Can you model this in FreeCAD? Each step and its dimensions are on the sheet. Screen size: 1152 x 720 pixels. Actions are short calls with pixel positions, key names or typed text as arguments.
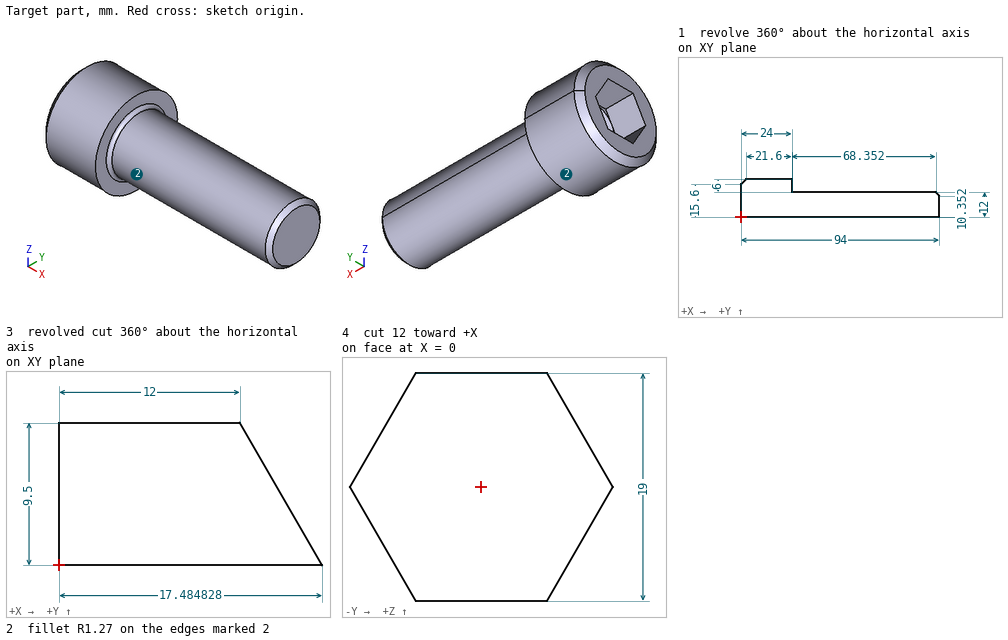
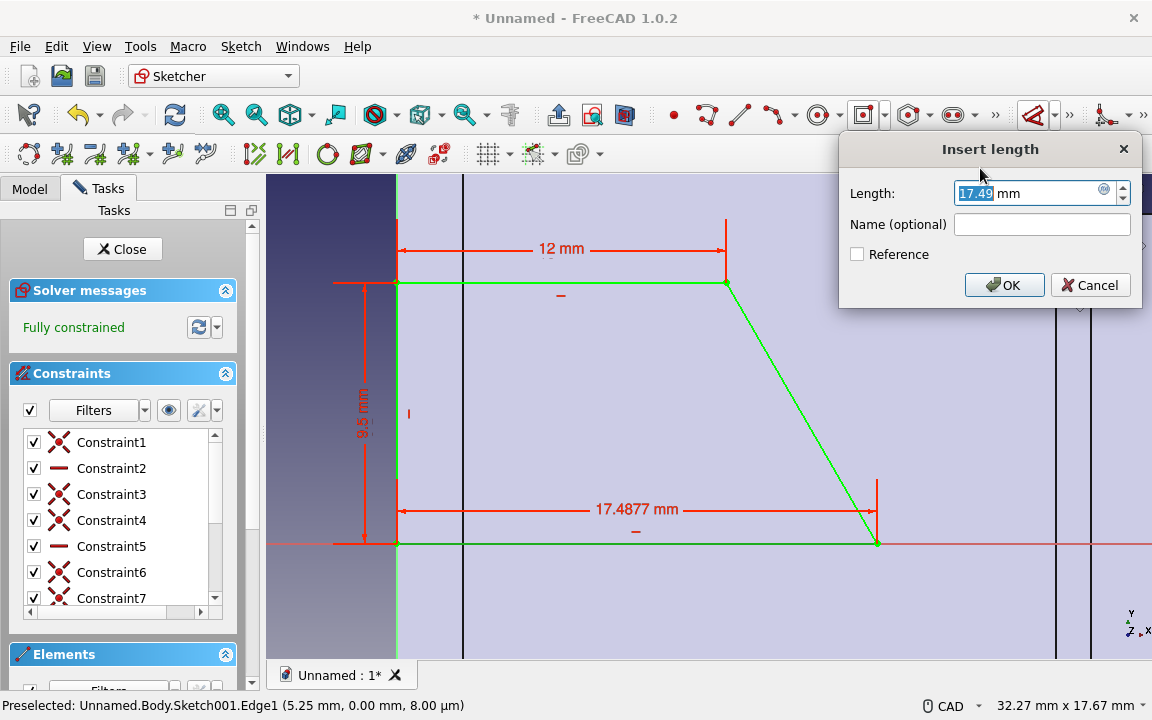
text(17.484828)
key(Return)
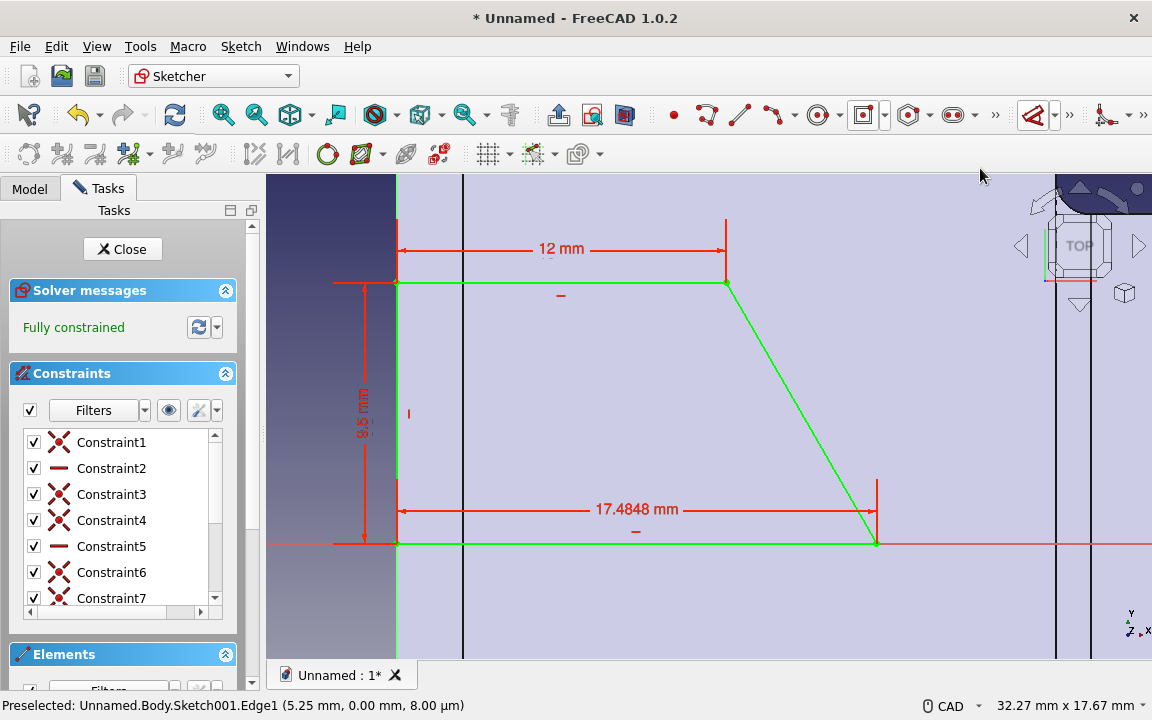
click(123, 249)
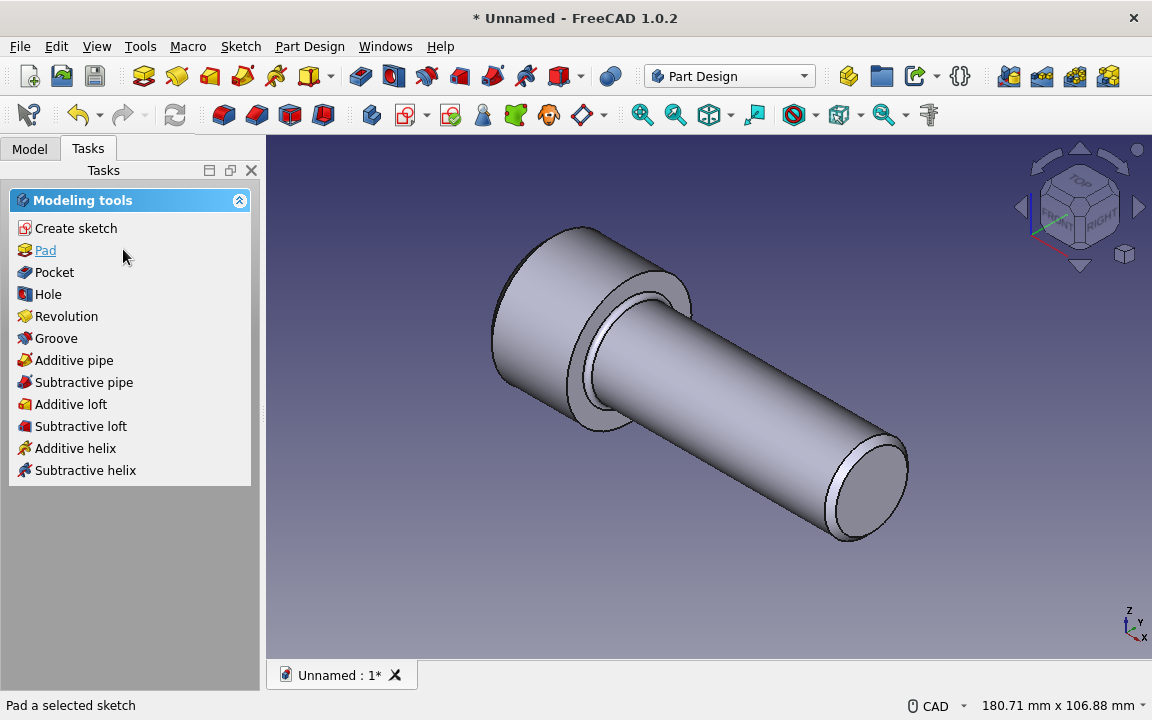
click(427, 76)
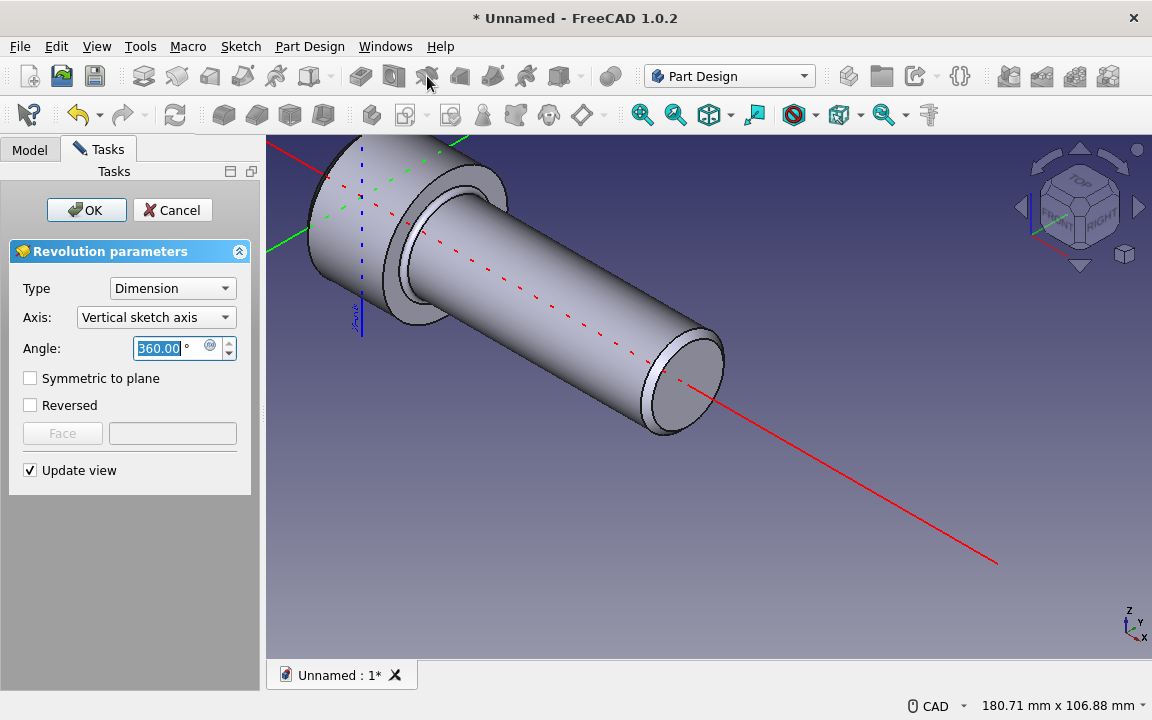
click(157, 318)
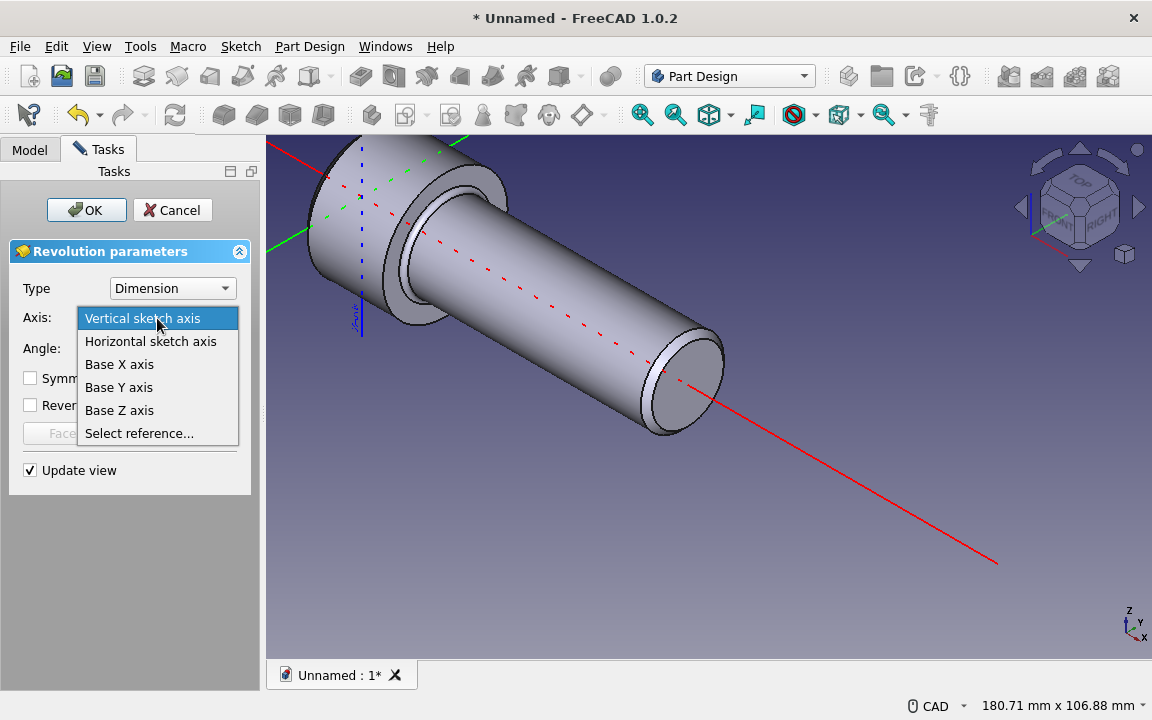
click(156, 342)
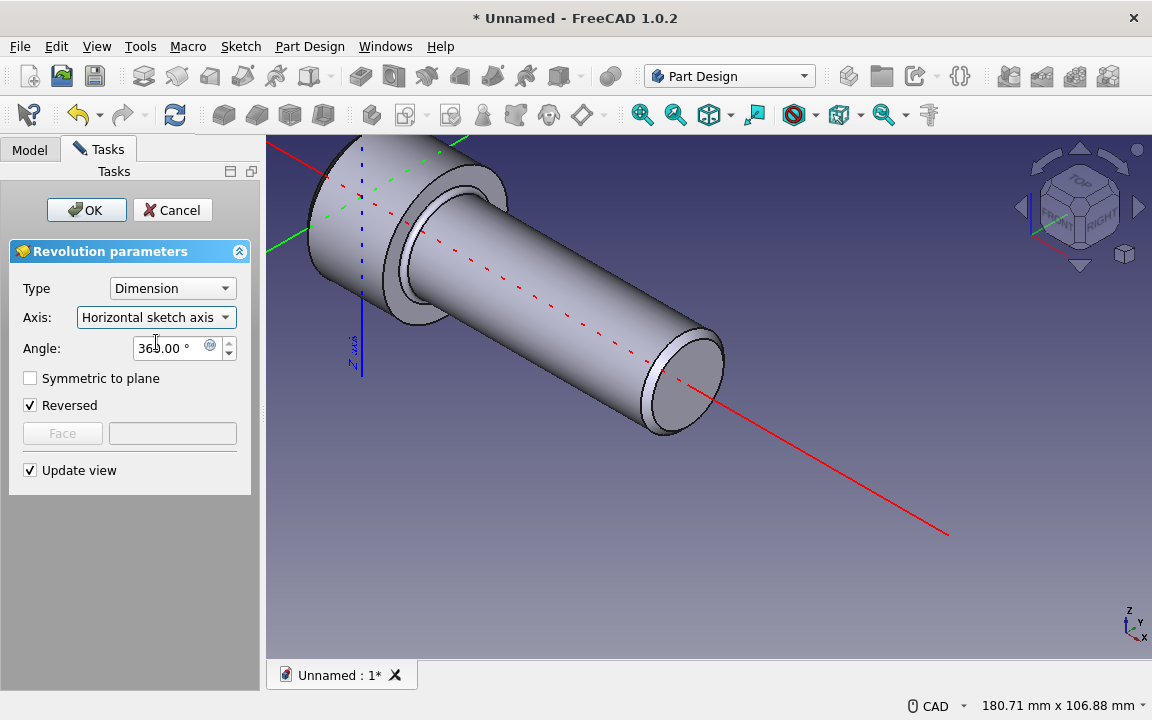
click(87, 210)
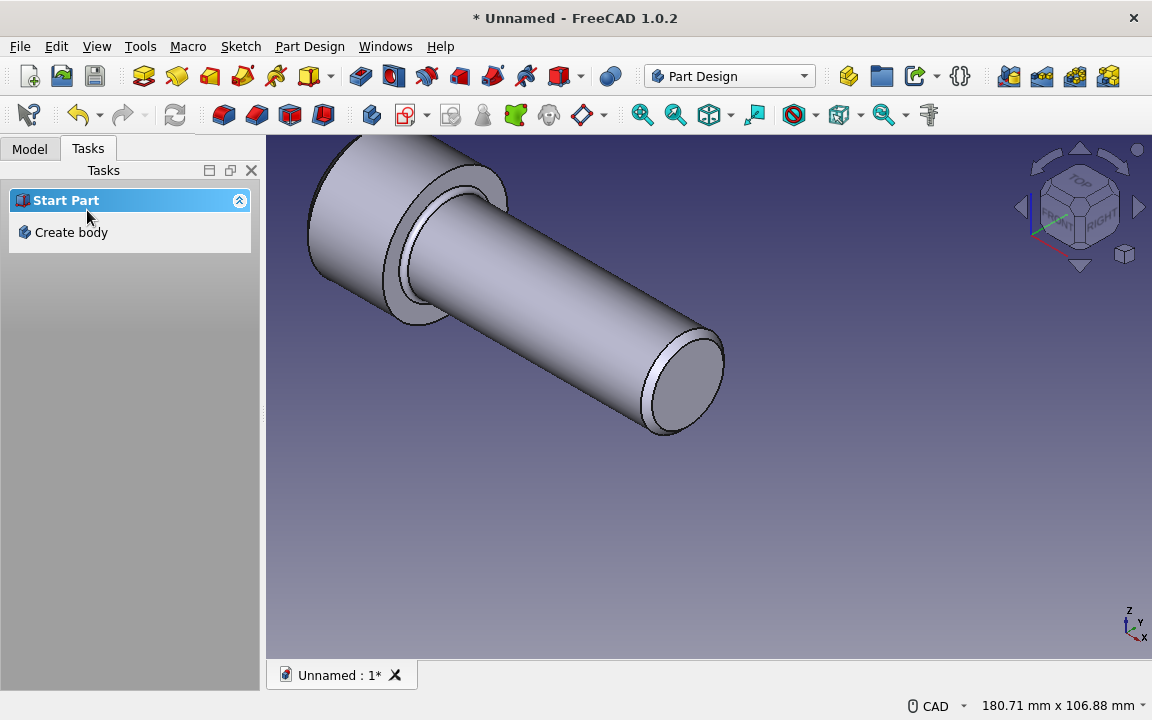
click(643, 116)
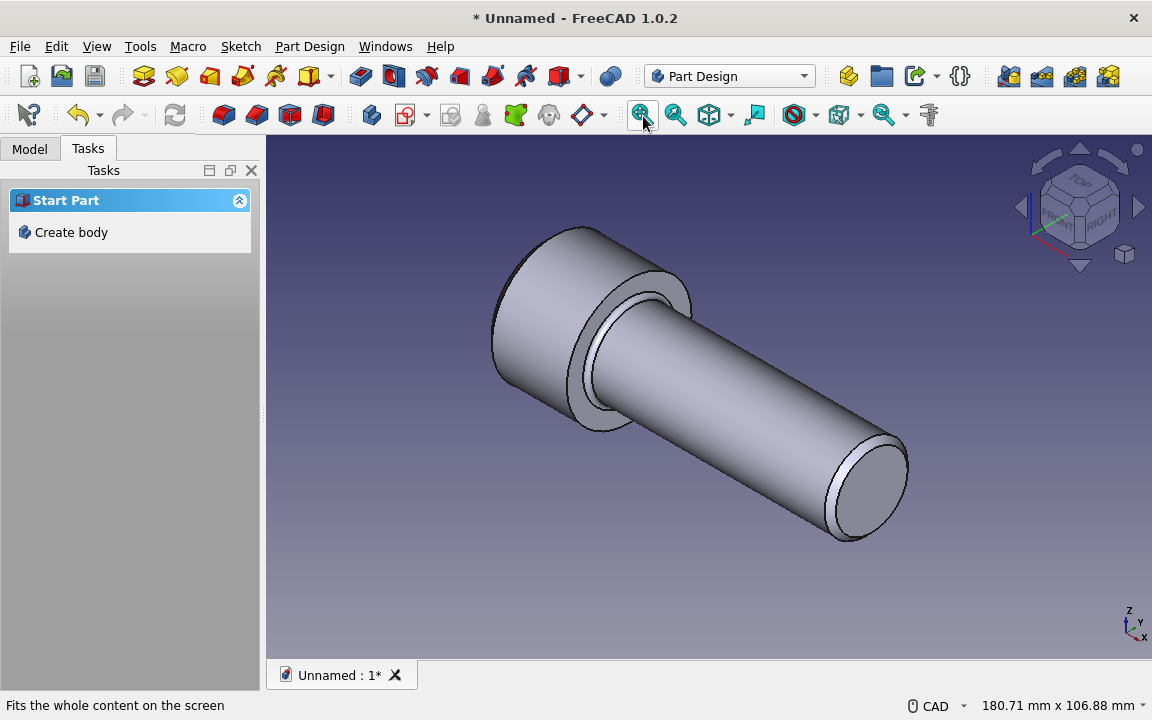
key(6)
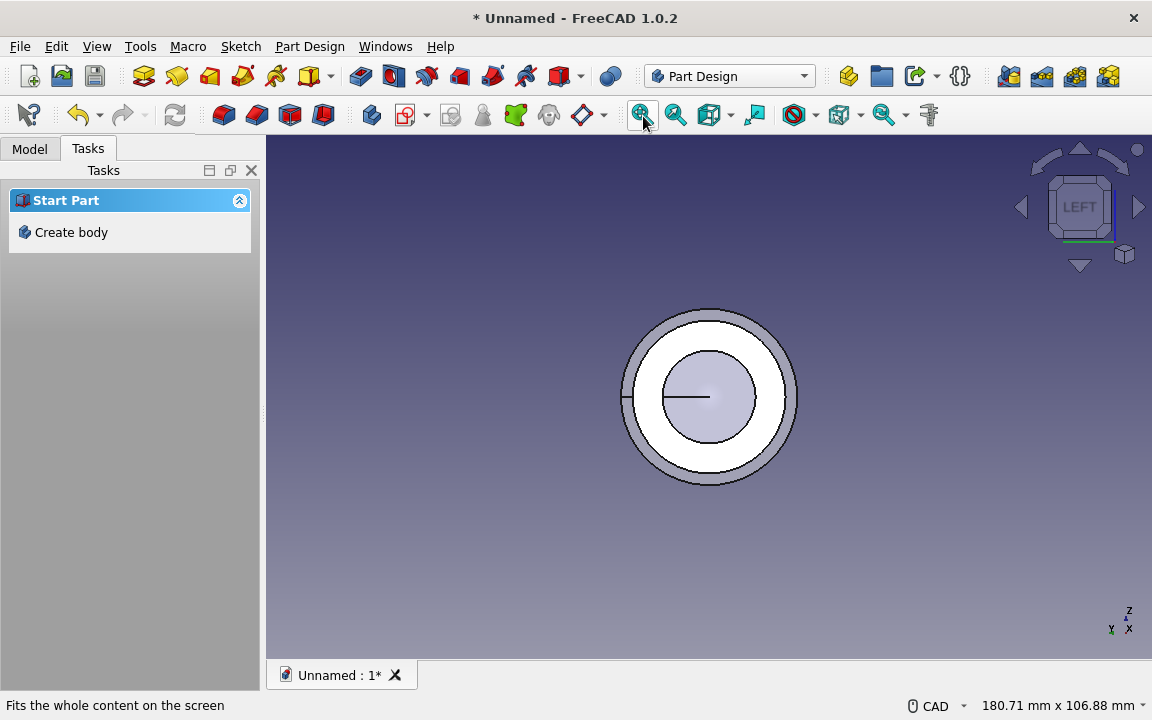
click(643, 116)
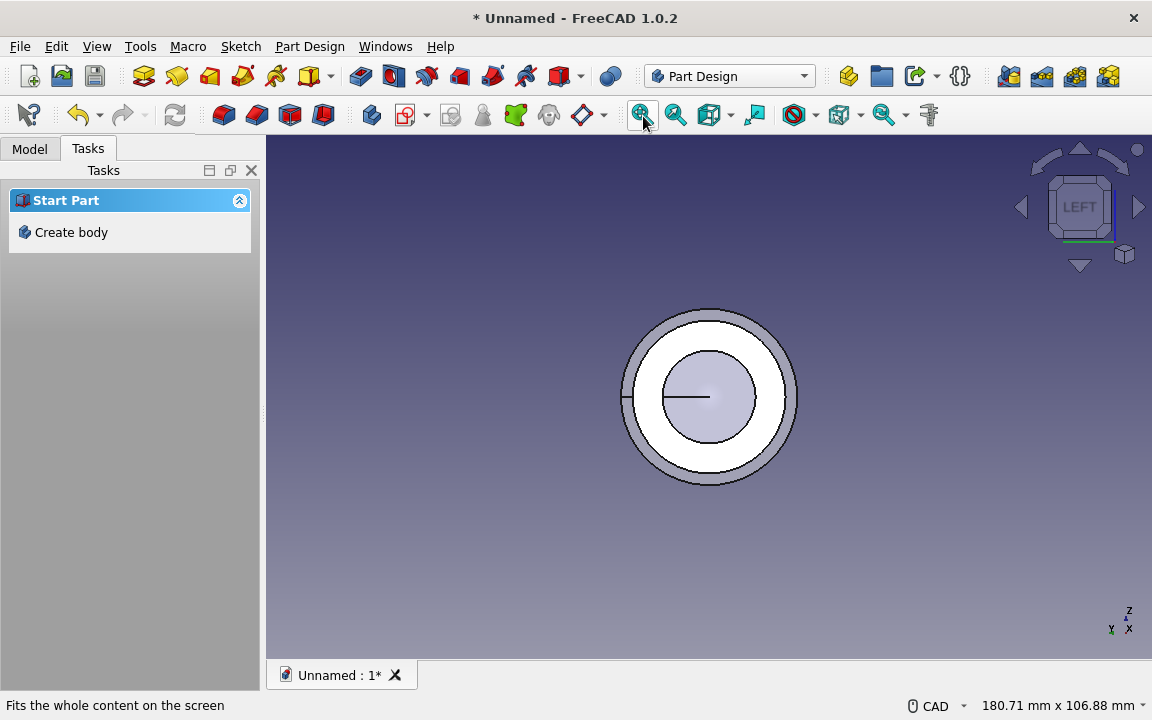
click(665, 352)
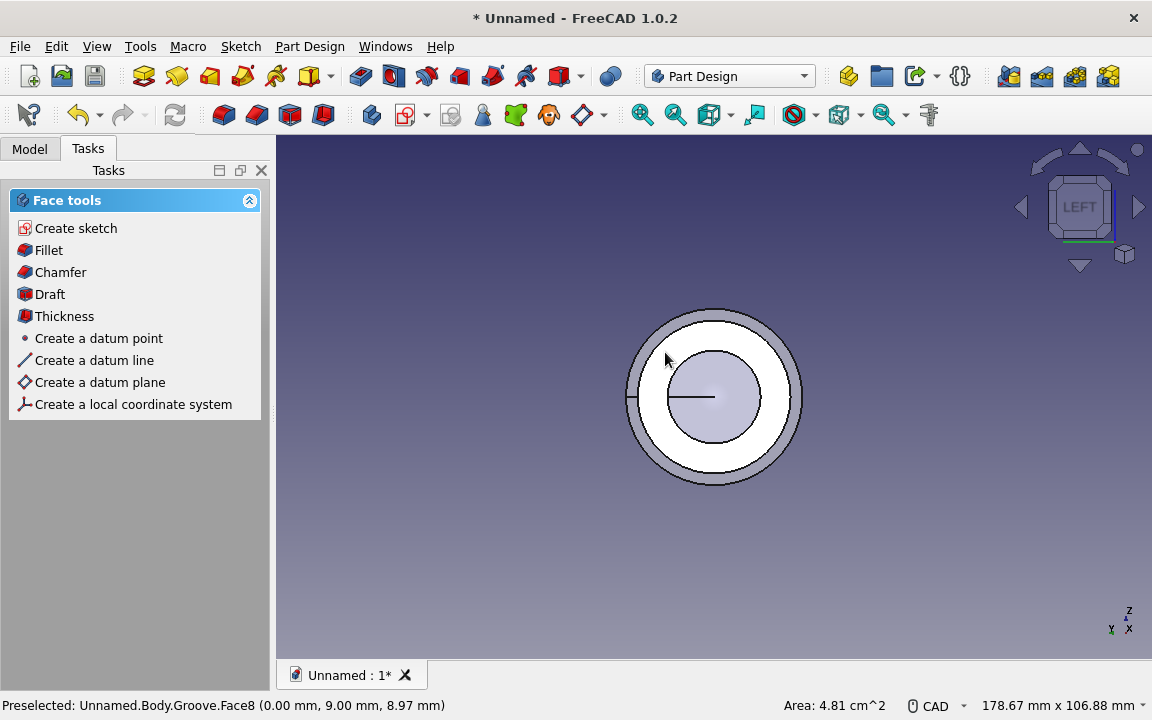
click(404, 116)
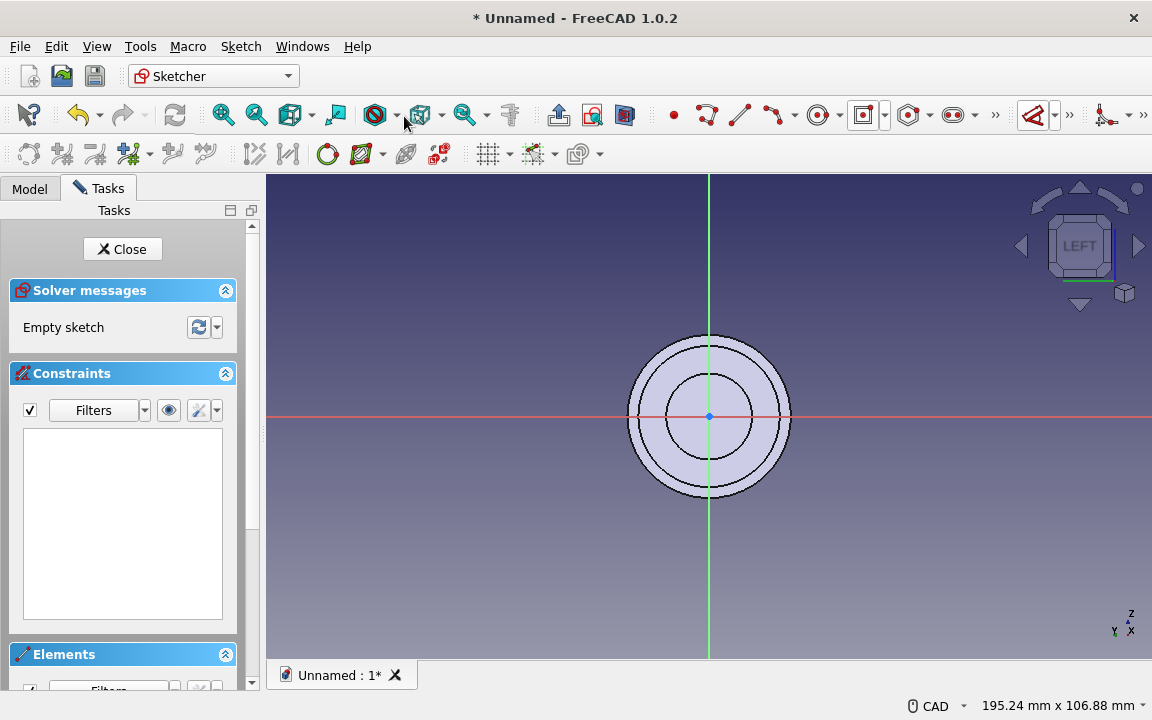
scroll(739, 416, up, 6)